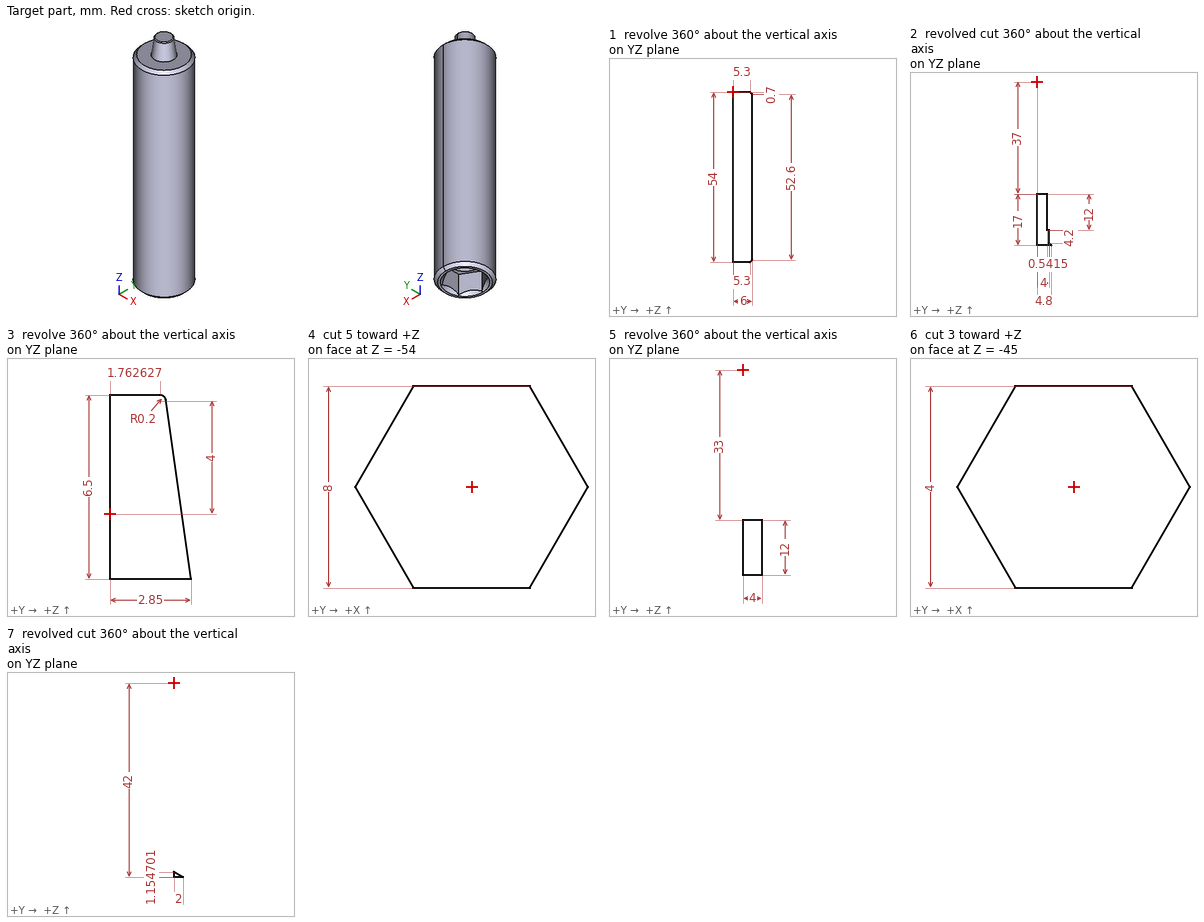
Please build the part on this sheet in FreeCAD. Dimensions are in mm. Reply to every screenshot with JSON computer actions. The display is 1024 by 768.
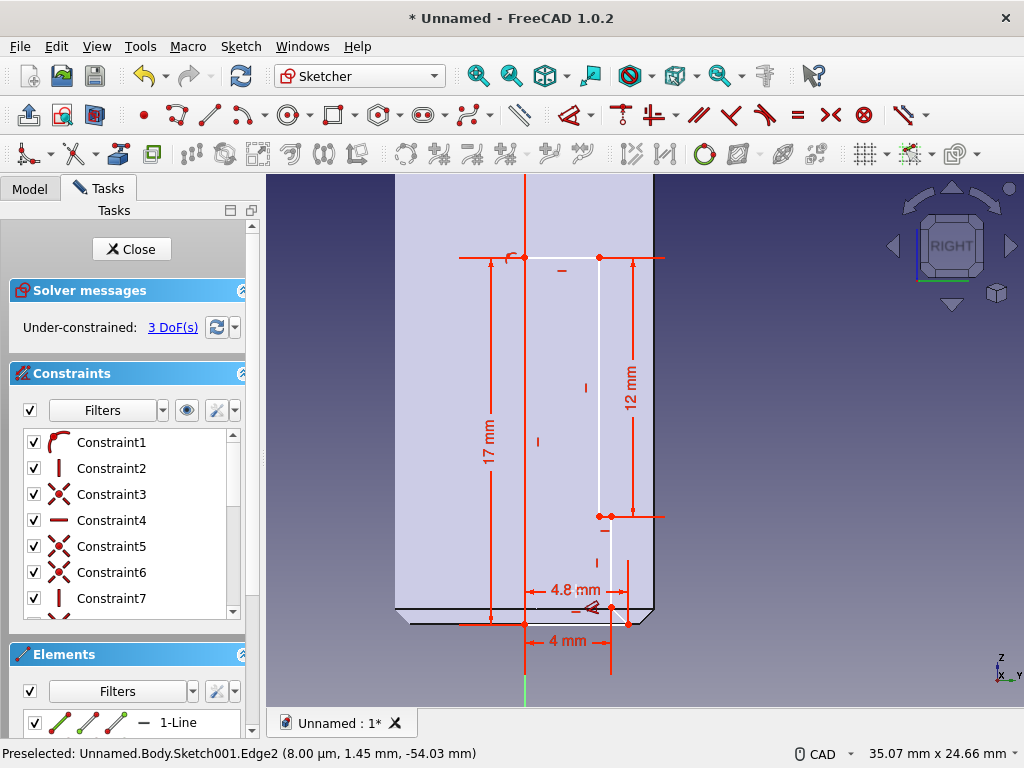
{"action": "left_click", "coordinate": [611, 581]}
{"action": "left_click", "coordinate": [645, 562]}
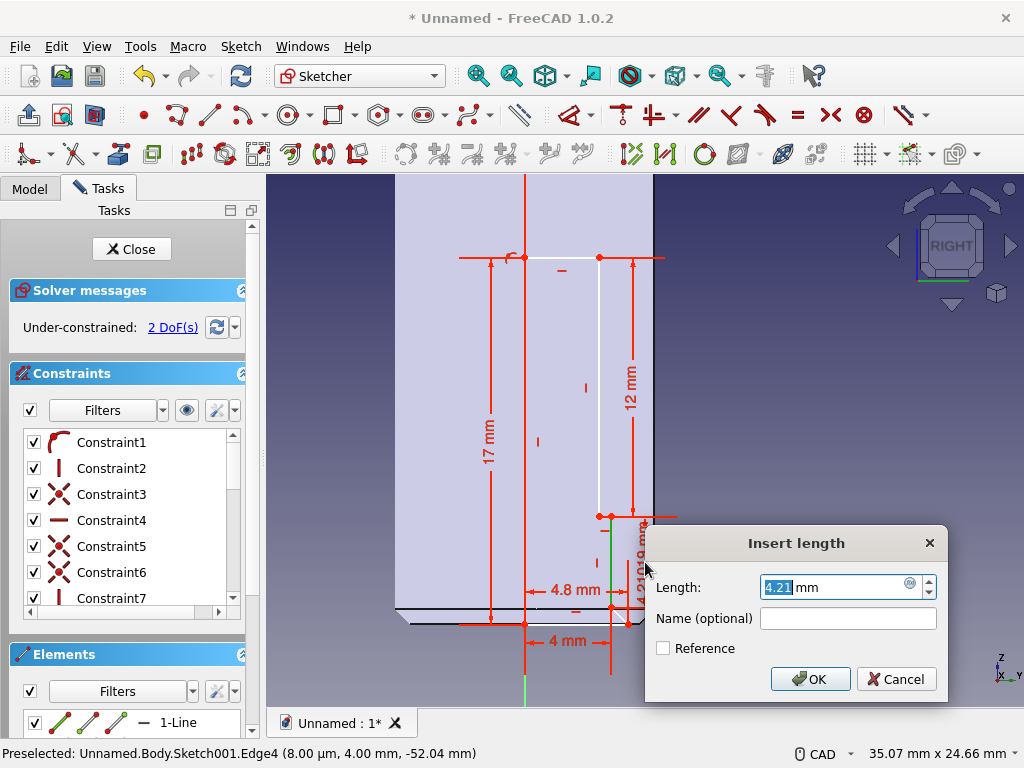
{"action": "type", "text": "4.2"}
{"action": "key", "text": "Return"}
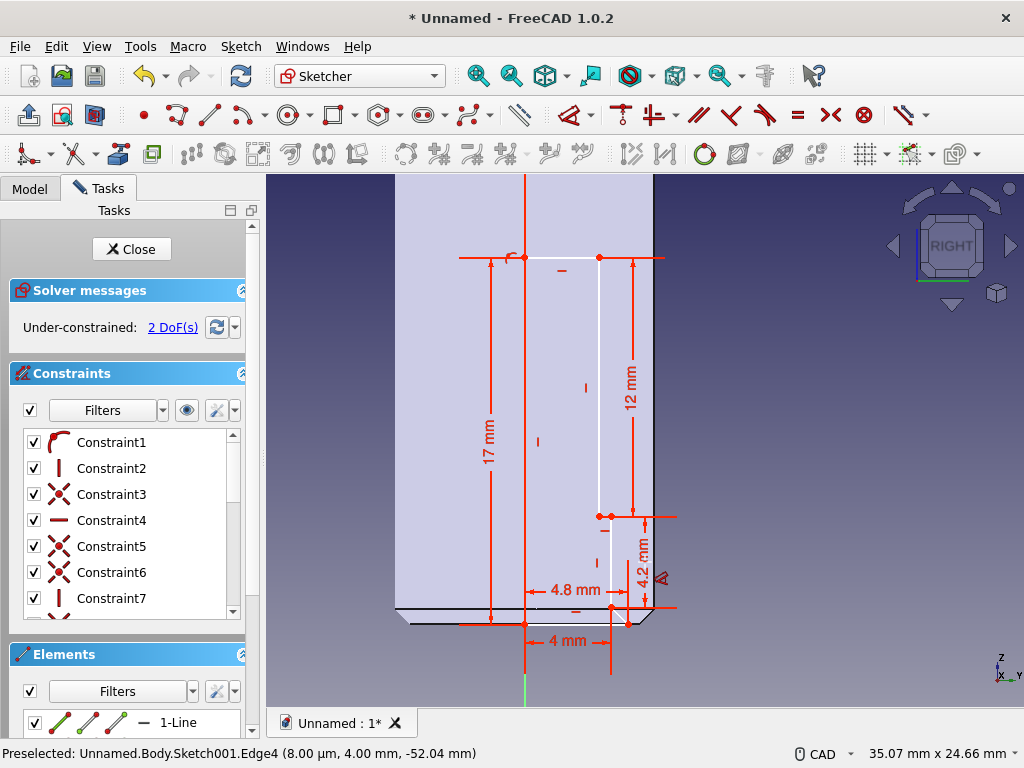
{"action": "left_click", "coordinate": [525, 258]}
{"action": "left_click", "coordinate": [491, 230]}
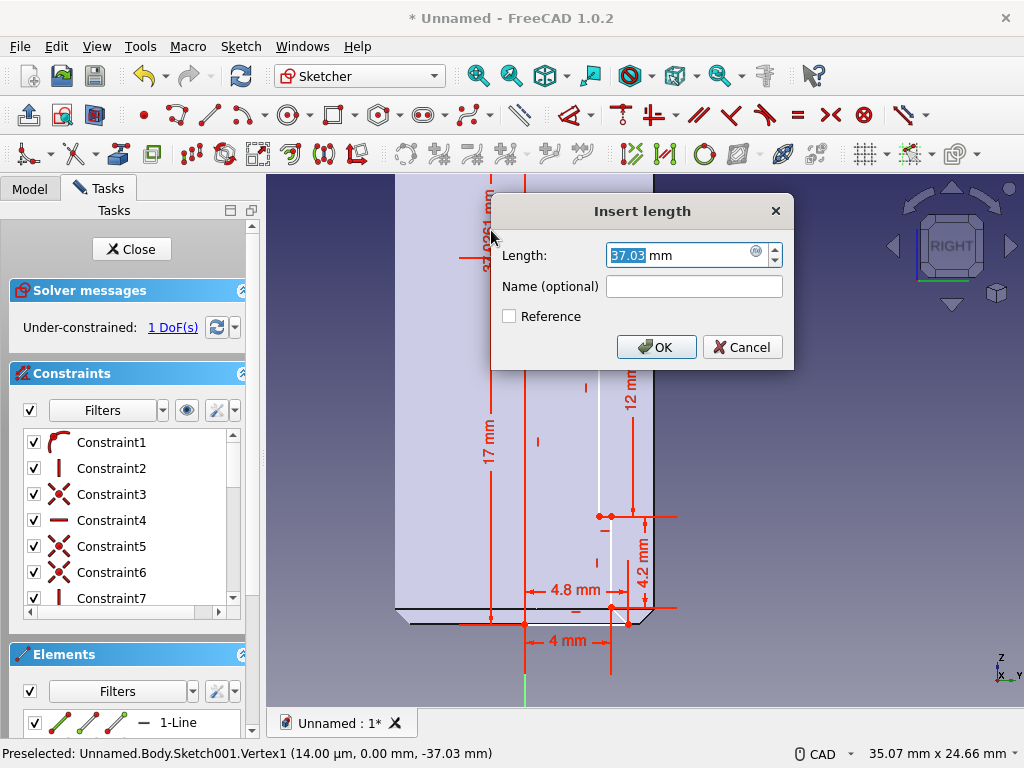
{"action": "type", "text": "37"}
{"action": "key", "text": "Return"}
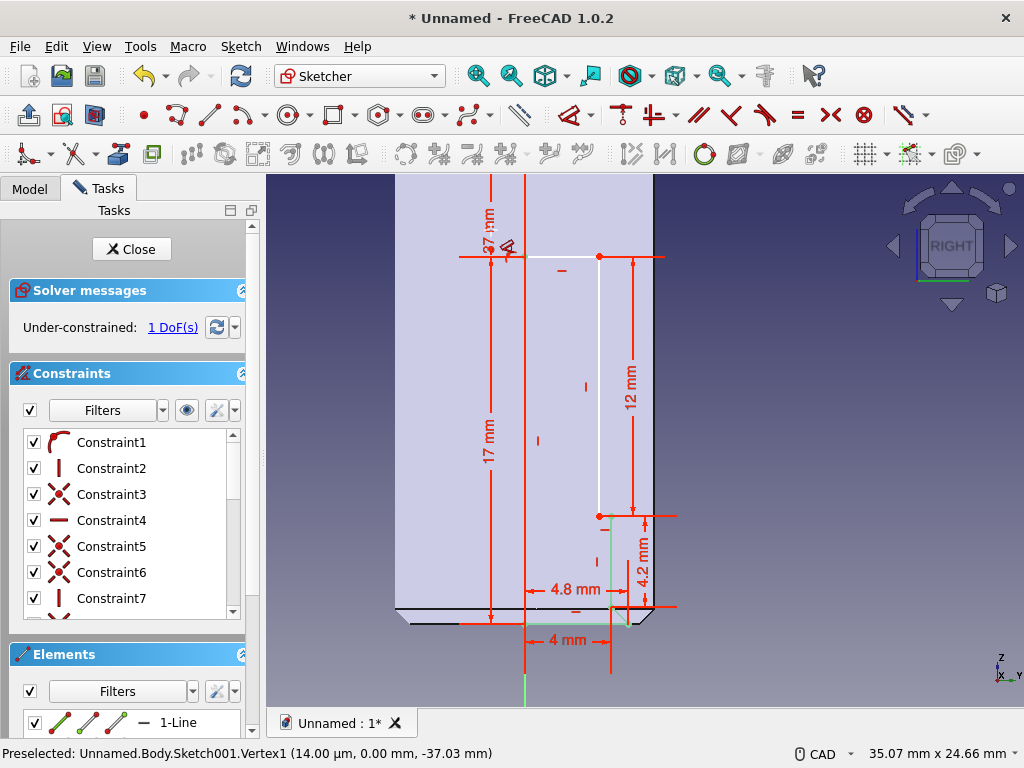
{"action": "scroll", "coordinate": [605, 516], "scroll_direction": "up", "scroll_amount": 7}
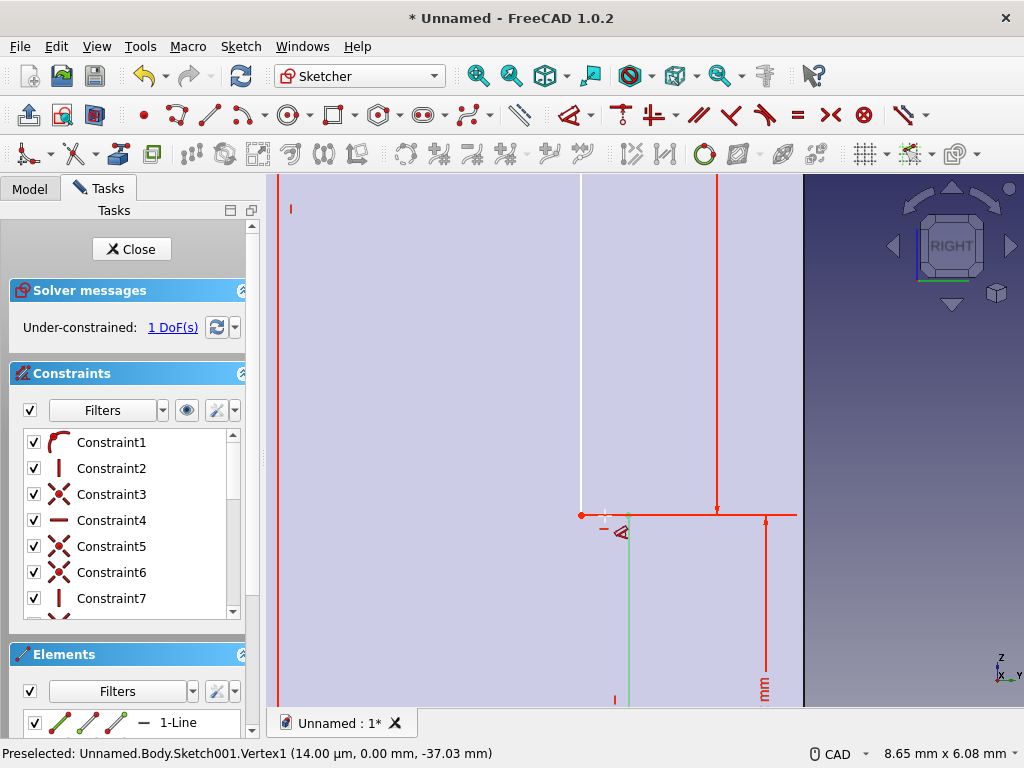
{"action": "left_click", "coordinate": [605, 515]}
{"action": "left_click", "coordinate": [605, 549]}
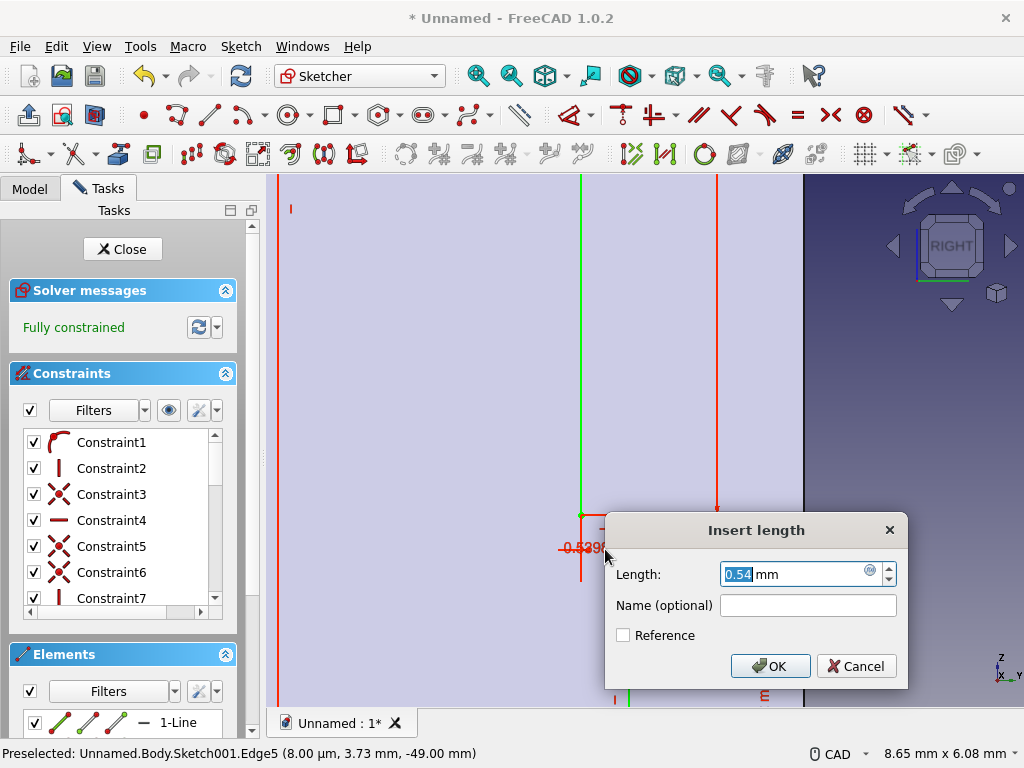
{"action": "type", "text": "0.5415"}
{"action": "key", "text": "Return"}
{"action": "key", "text": "Escape"}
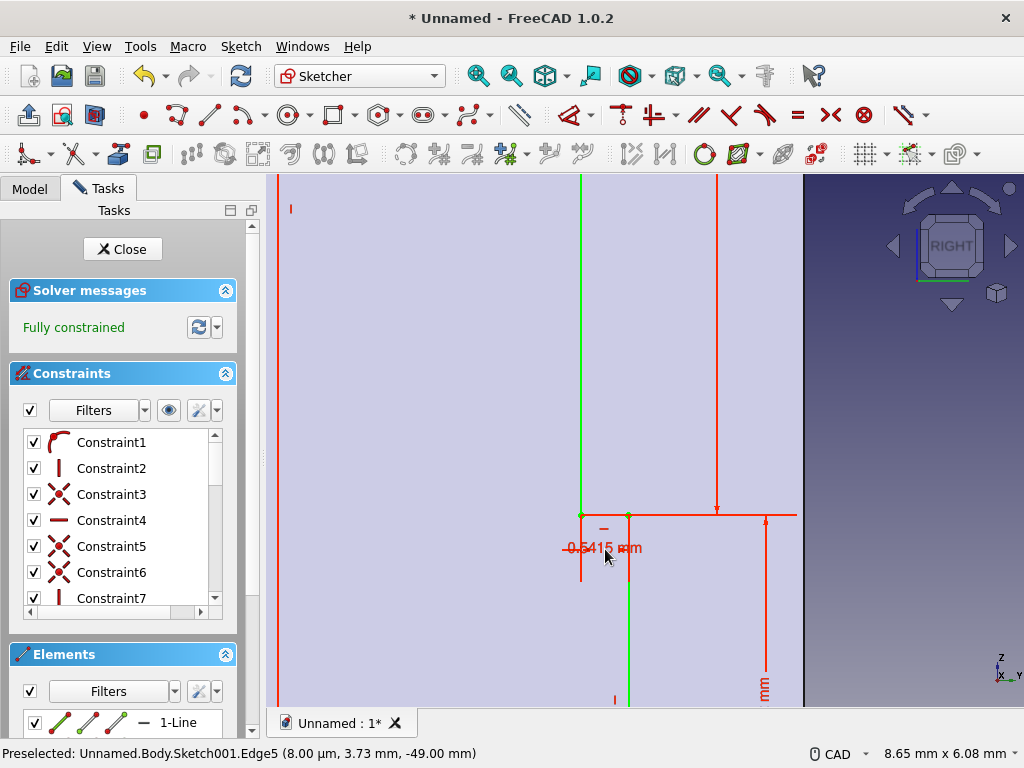
{"action": "left_click", "coordinate": [123, 249]}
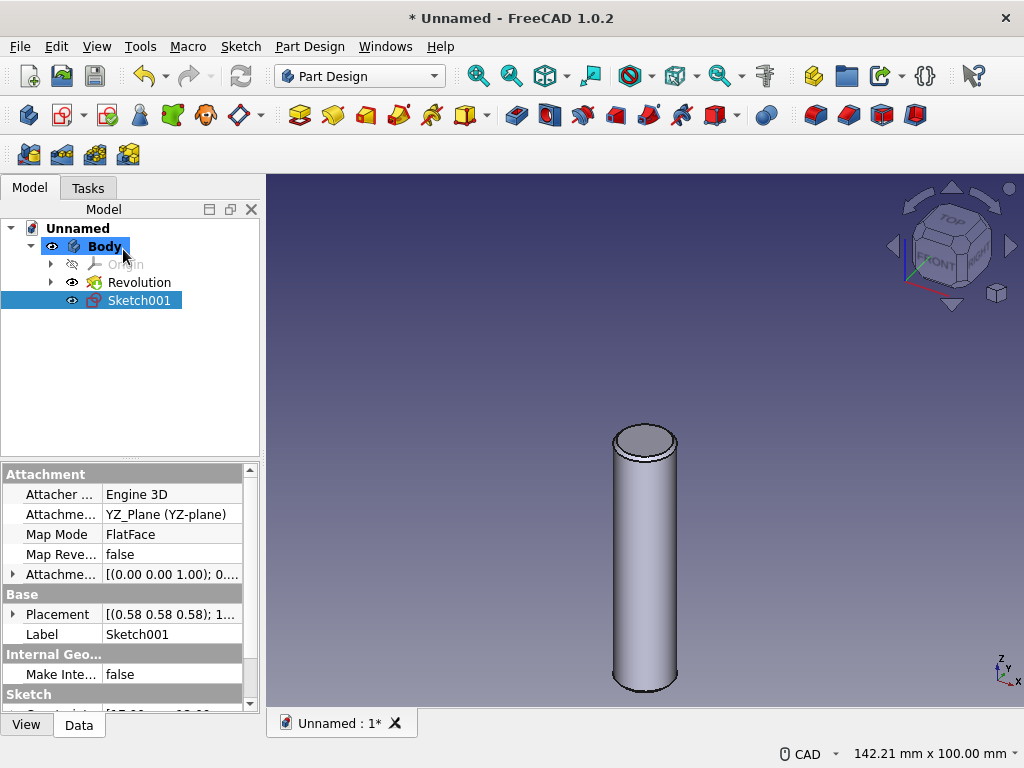
{"action": "left_click", "coordinate": [583, 116]}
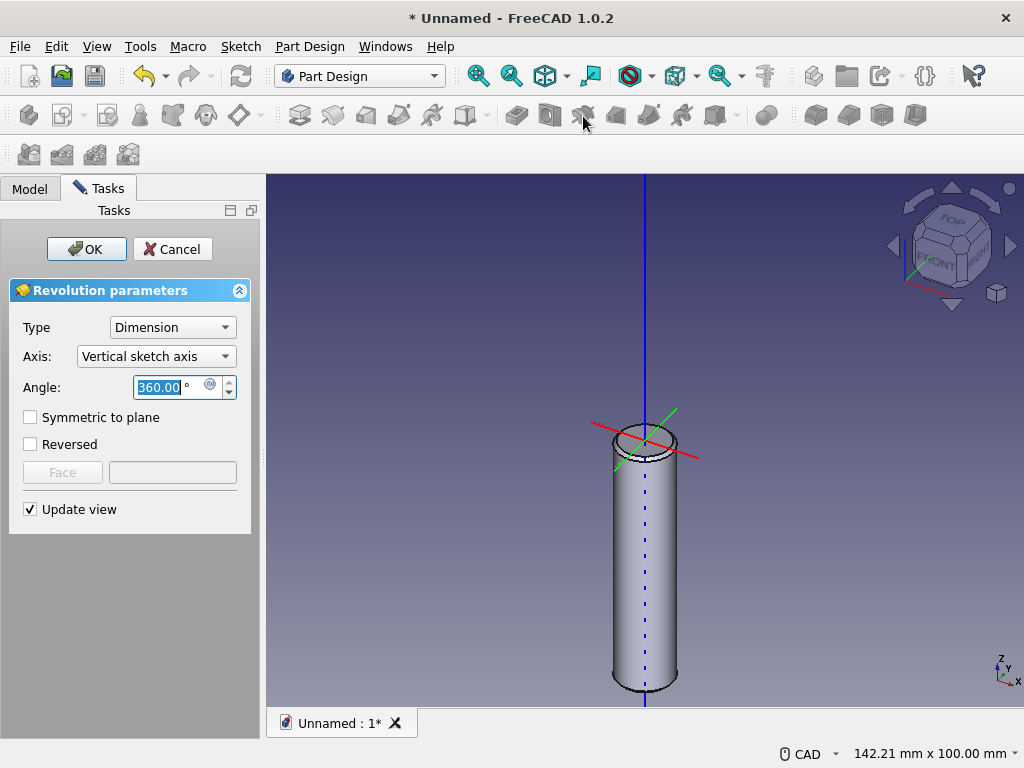
{"action": "left_click", "coordinate": [87, 249]}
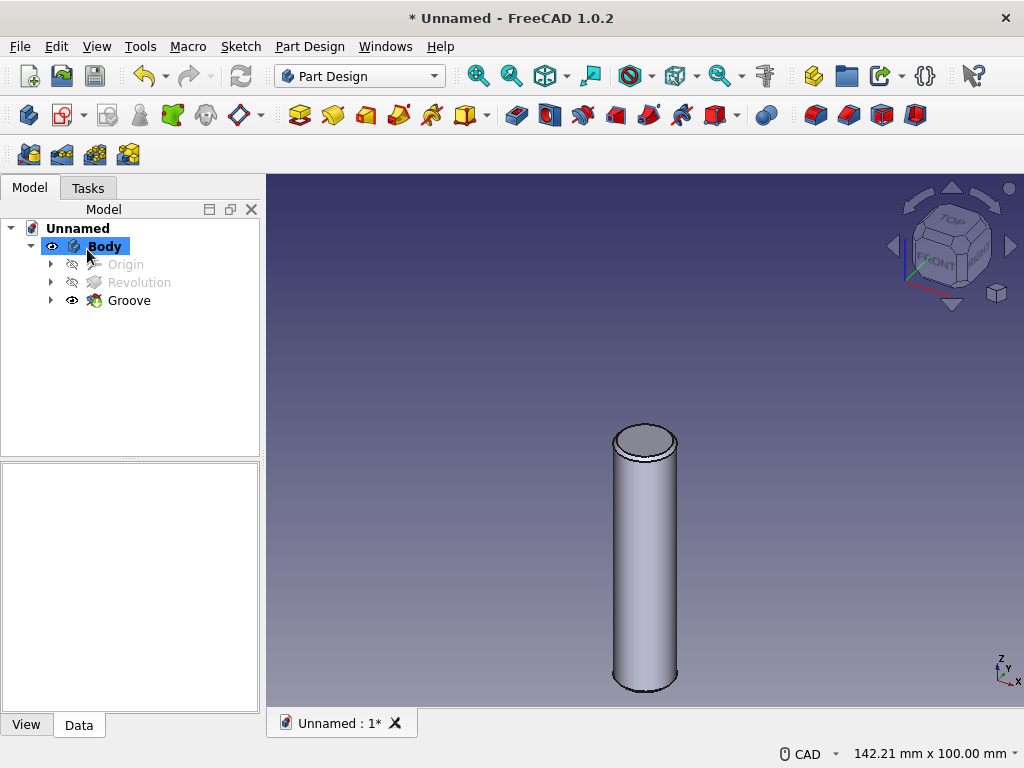
{"action": "left_click", "coordinate": [62, 116]}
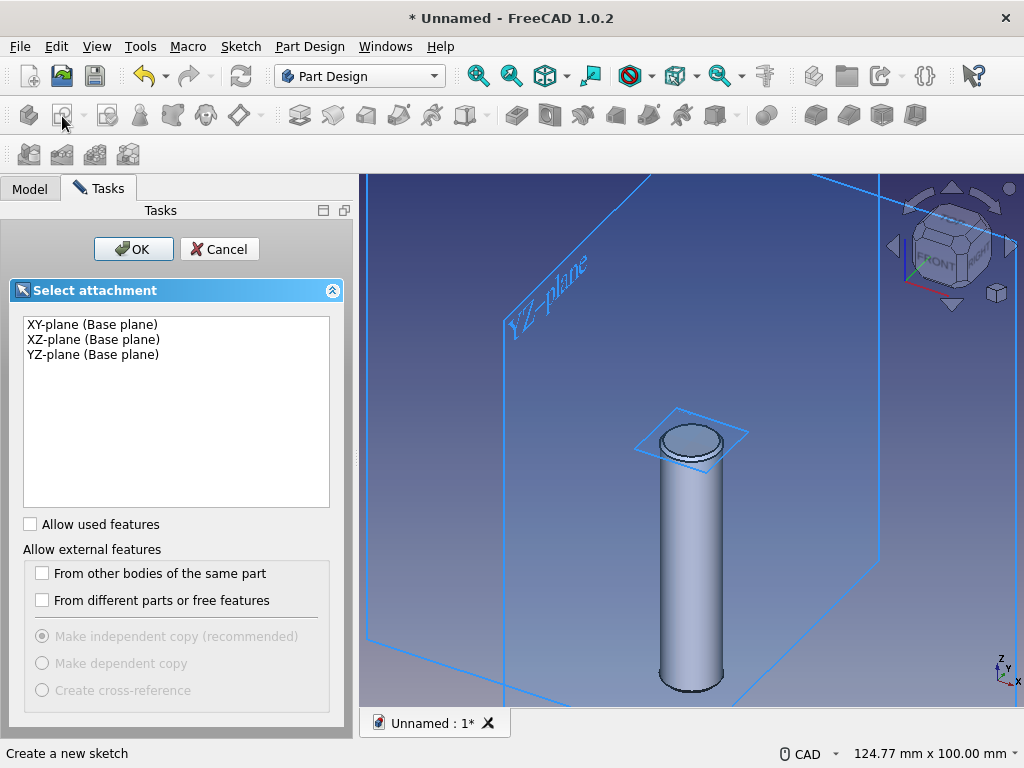
{"action": "left_click", "coordinate": [84, 354]}